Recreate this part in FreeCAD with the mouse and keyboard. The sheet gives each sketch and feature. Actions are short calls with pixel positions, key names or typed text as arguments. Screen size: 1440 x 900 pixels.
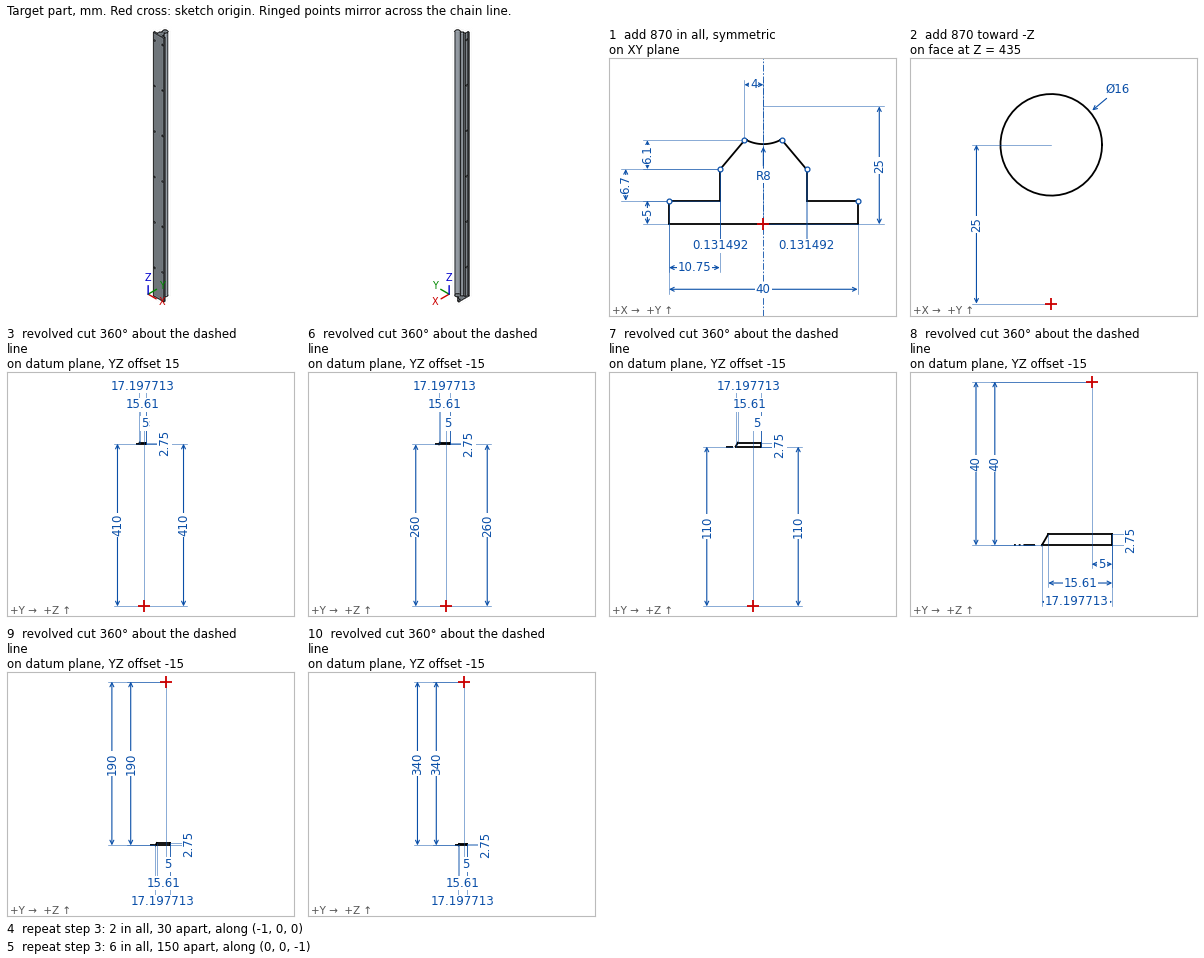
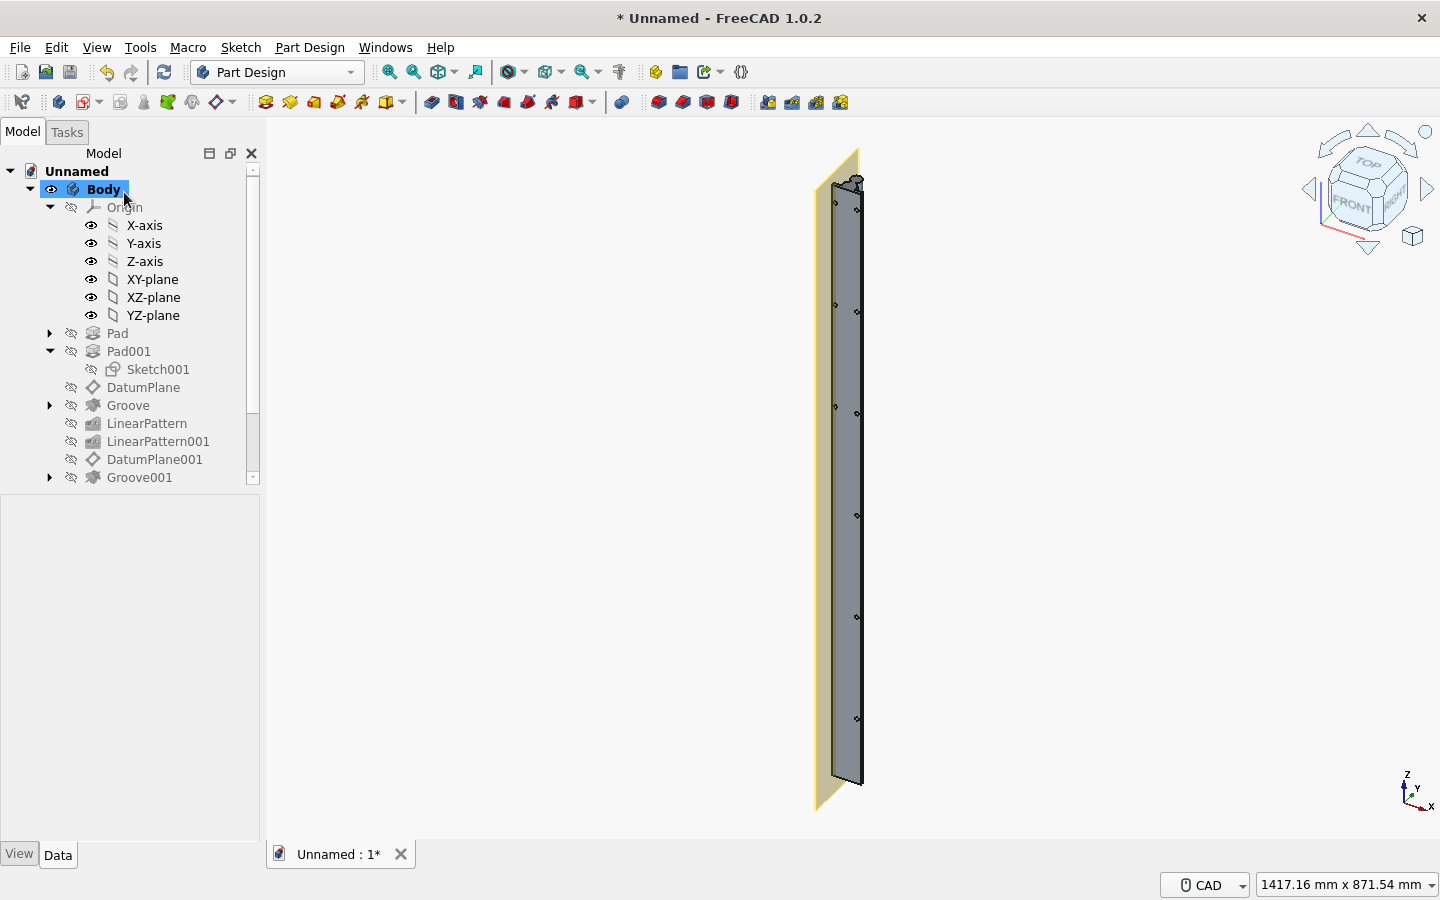
scroll(100, 329, down, 3)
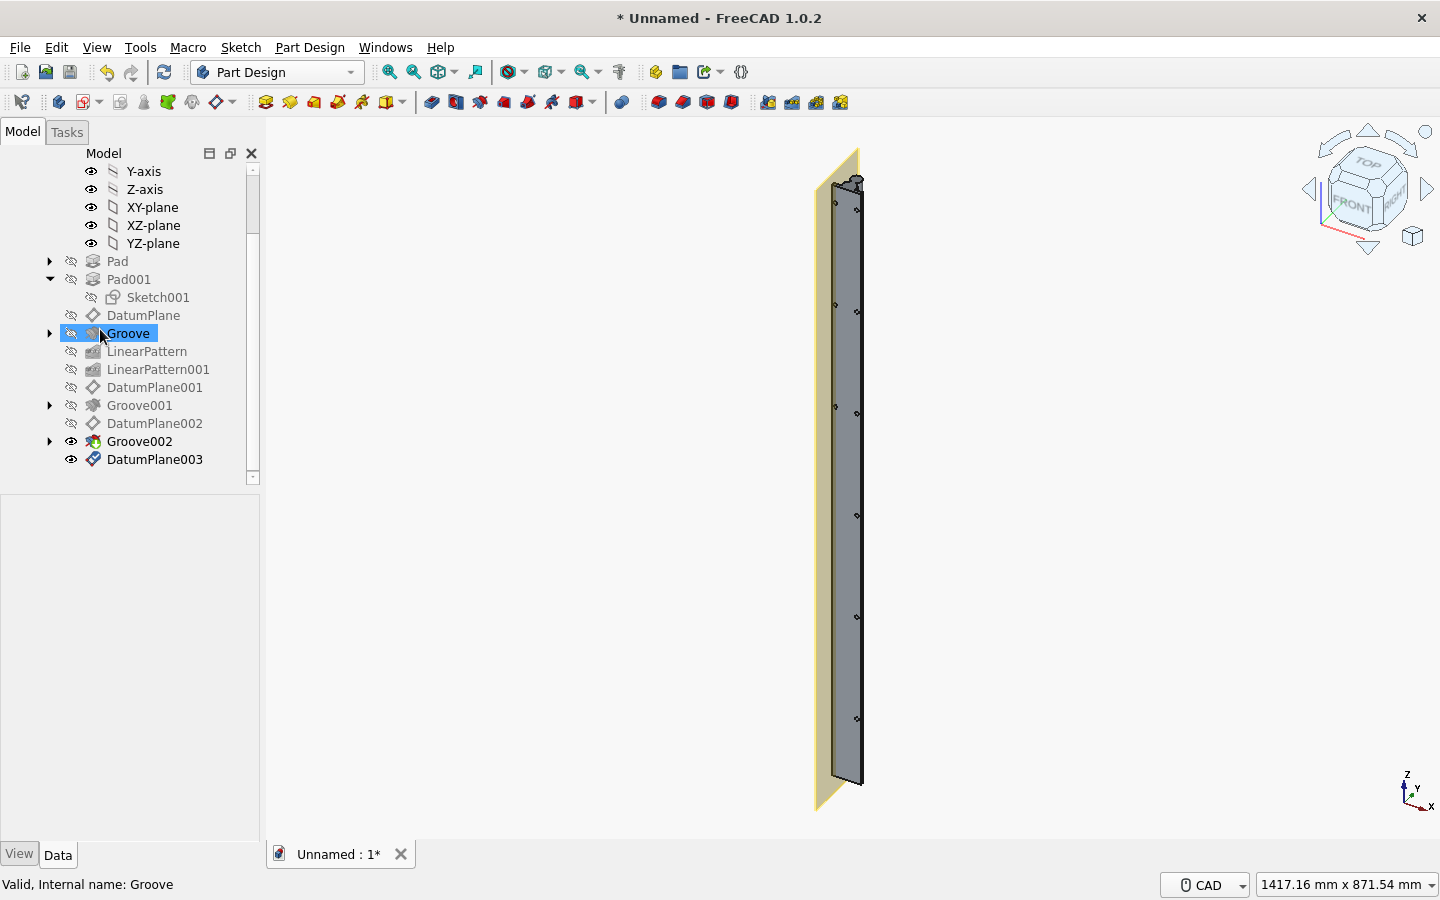
click(116, 459)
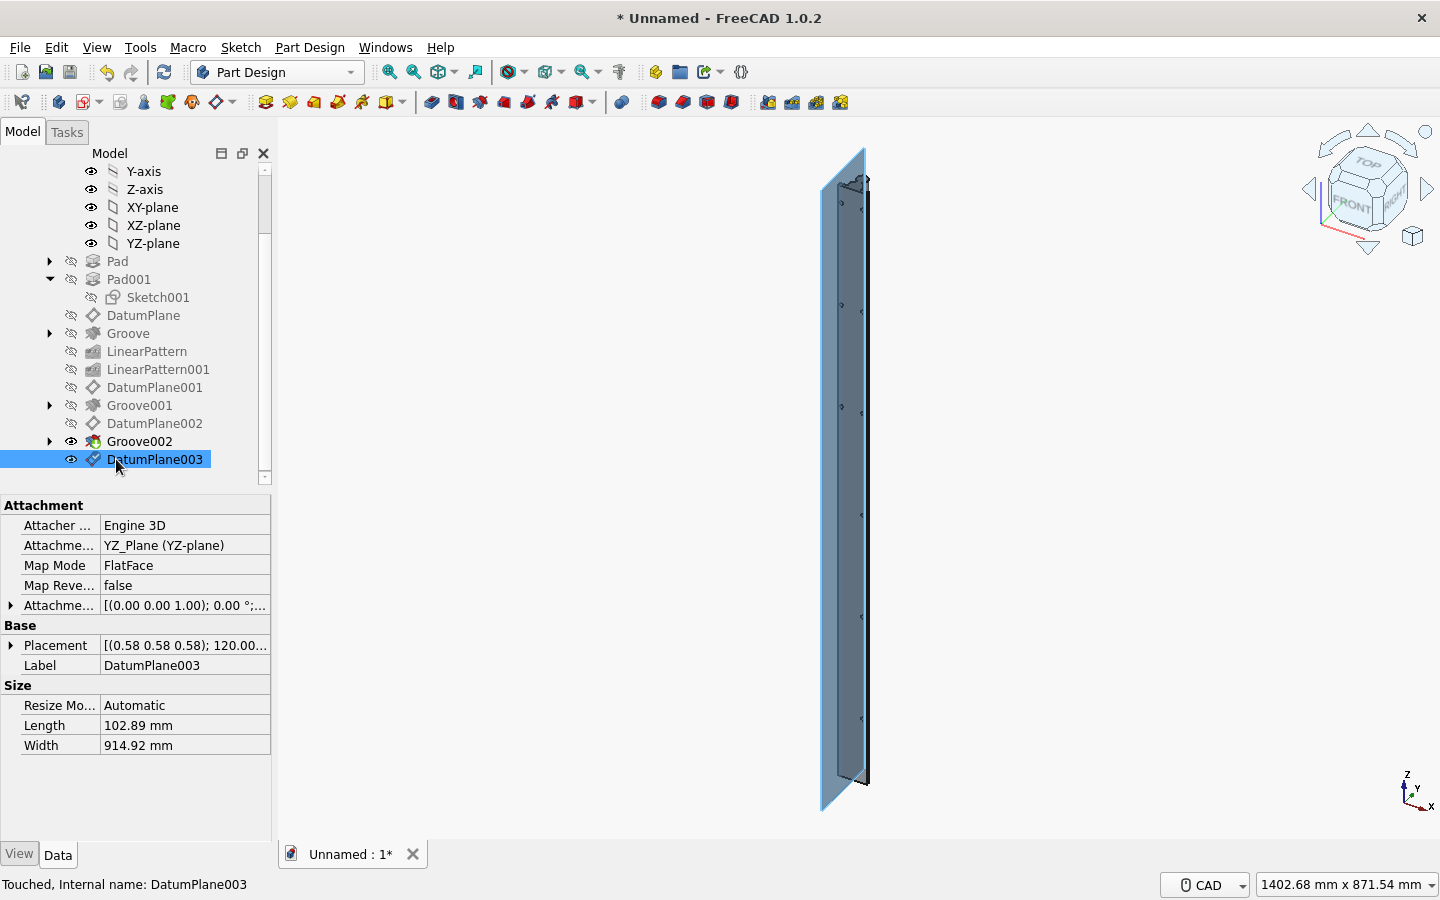
click(84, 102)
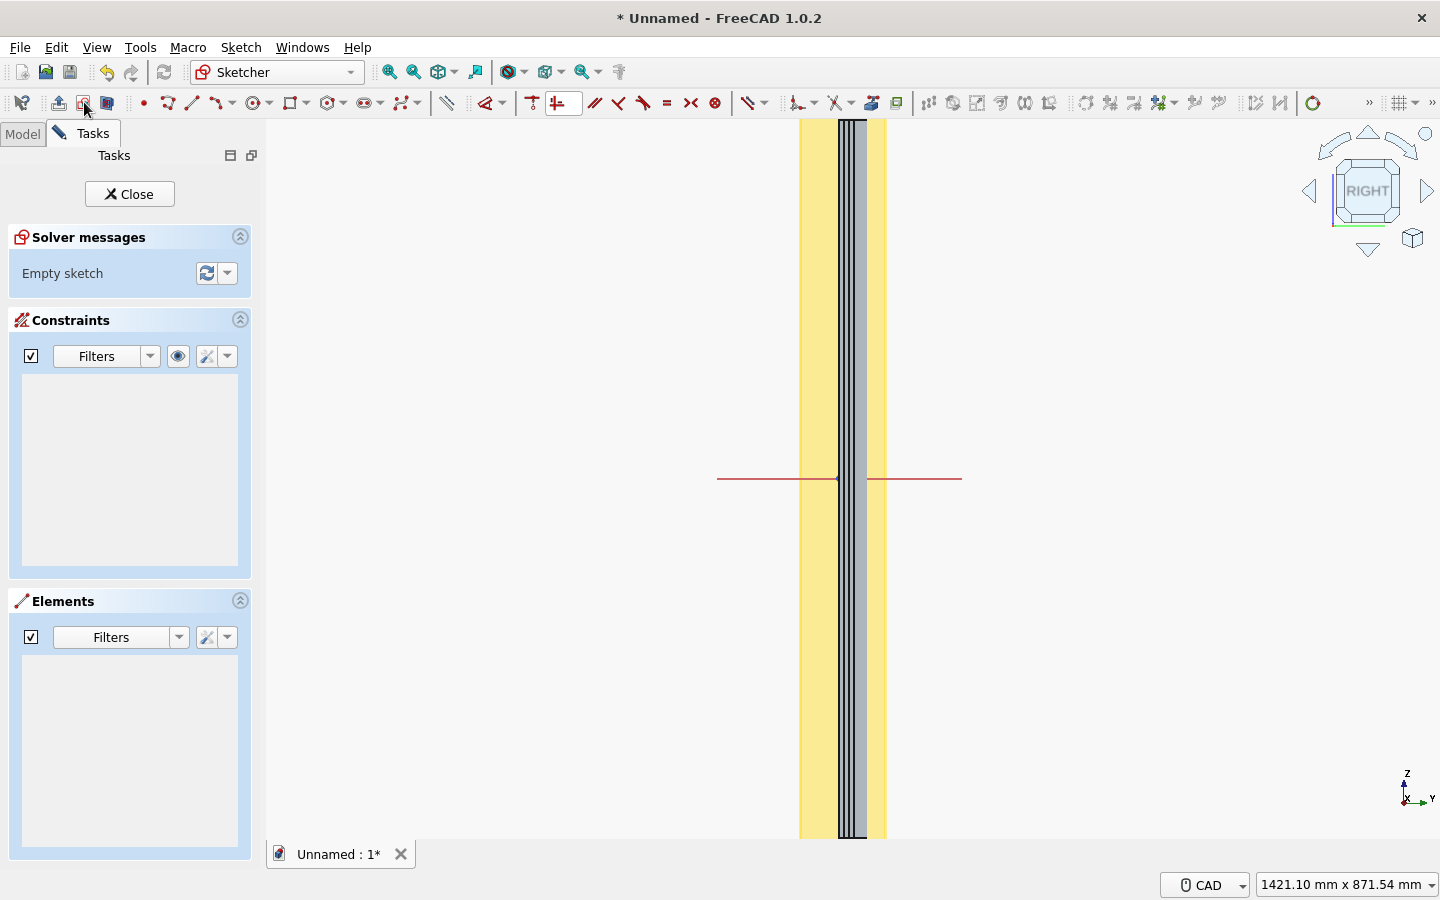
click(108, 104)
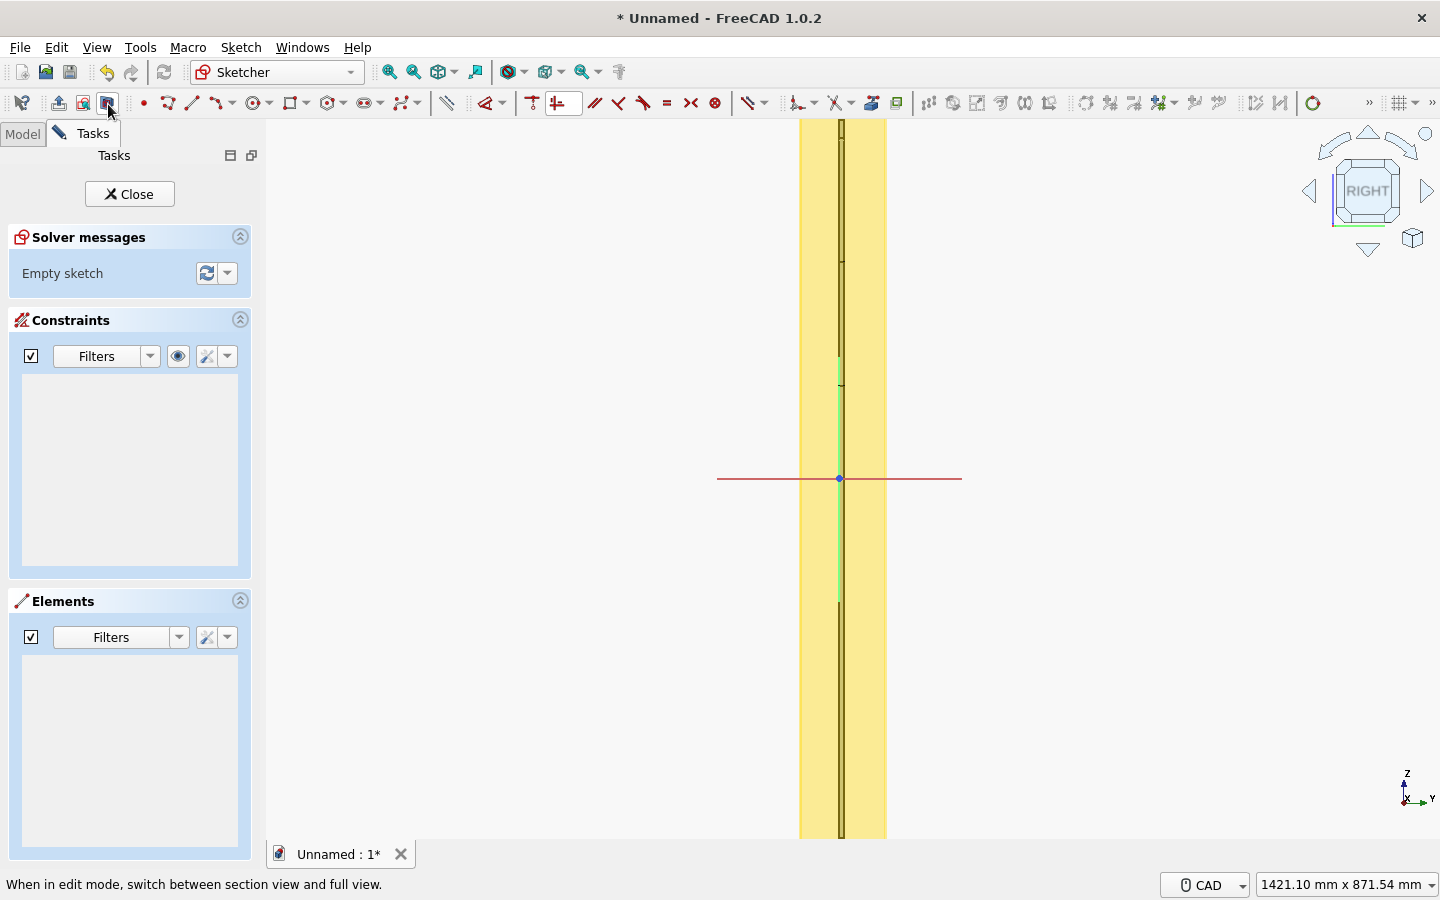
scroll(838, 497, up, 13)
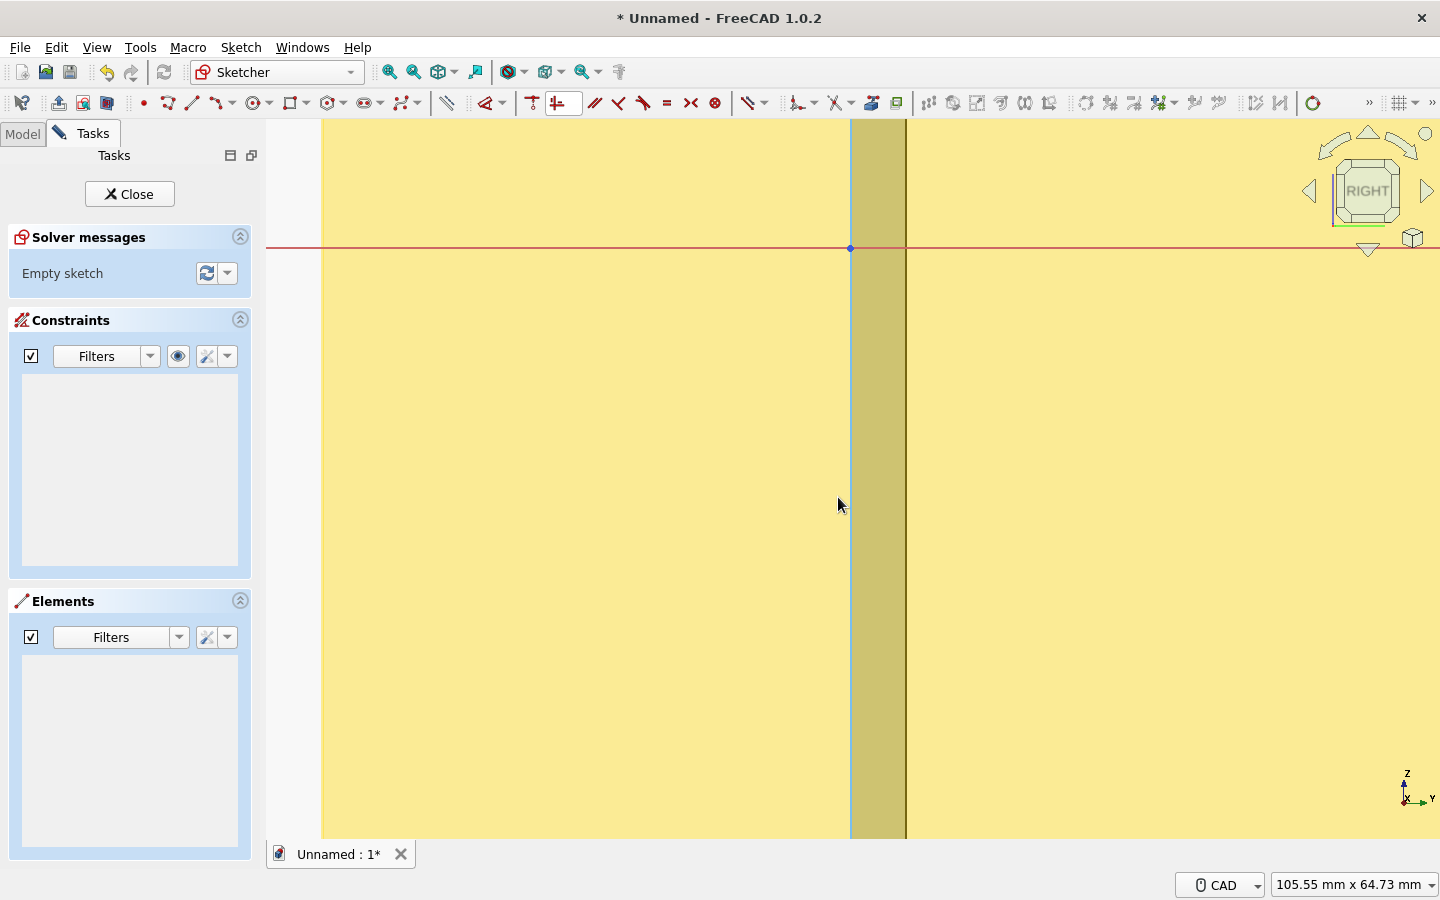
click(168, 104)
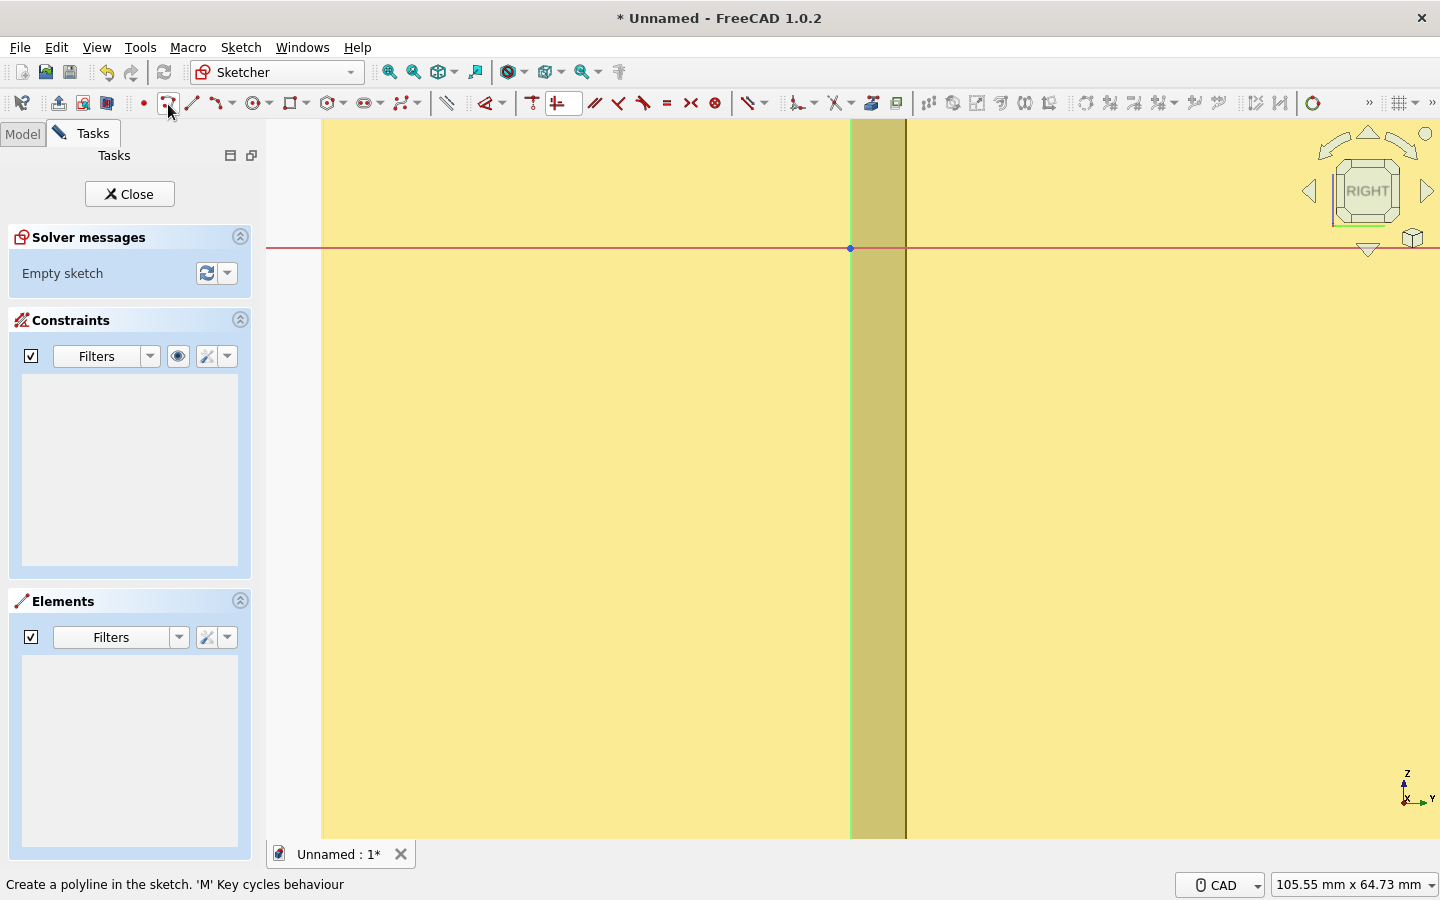
click(906, 662)
click(733, 662)
click(715, 693)
click(906, 693)
click(906, 663)